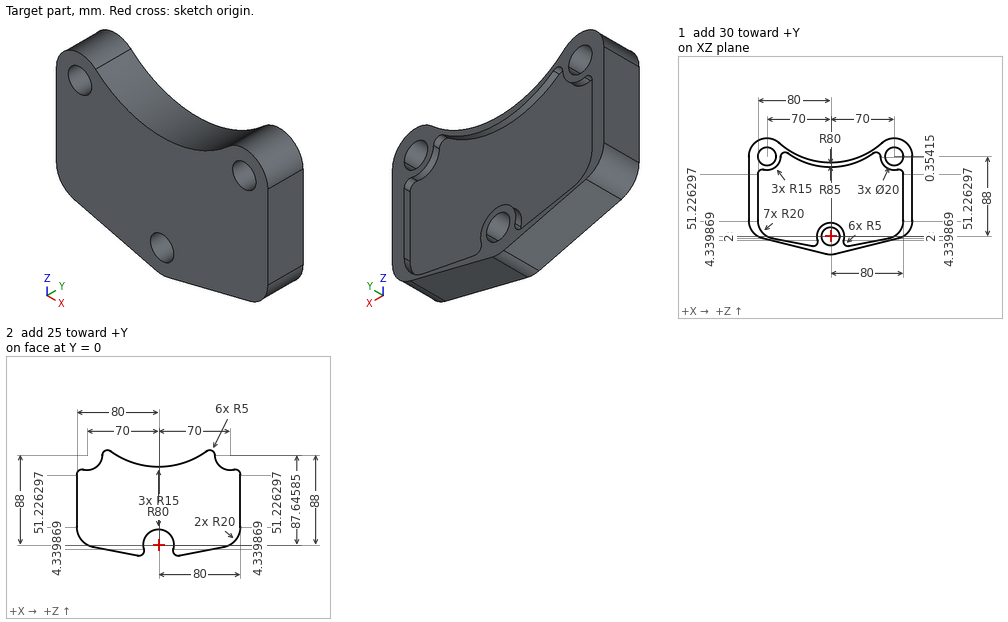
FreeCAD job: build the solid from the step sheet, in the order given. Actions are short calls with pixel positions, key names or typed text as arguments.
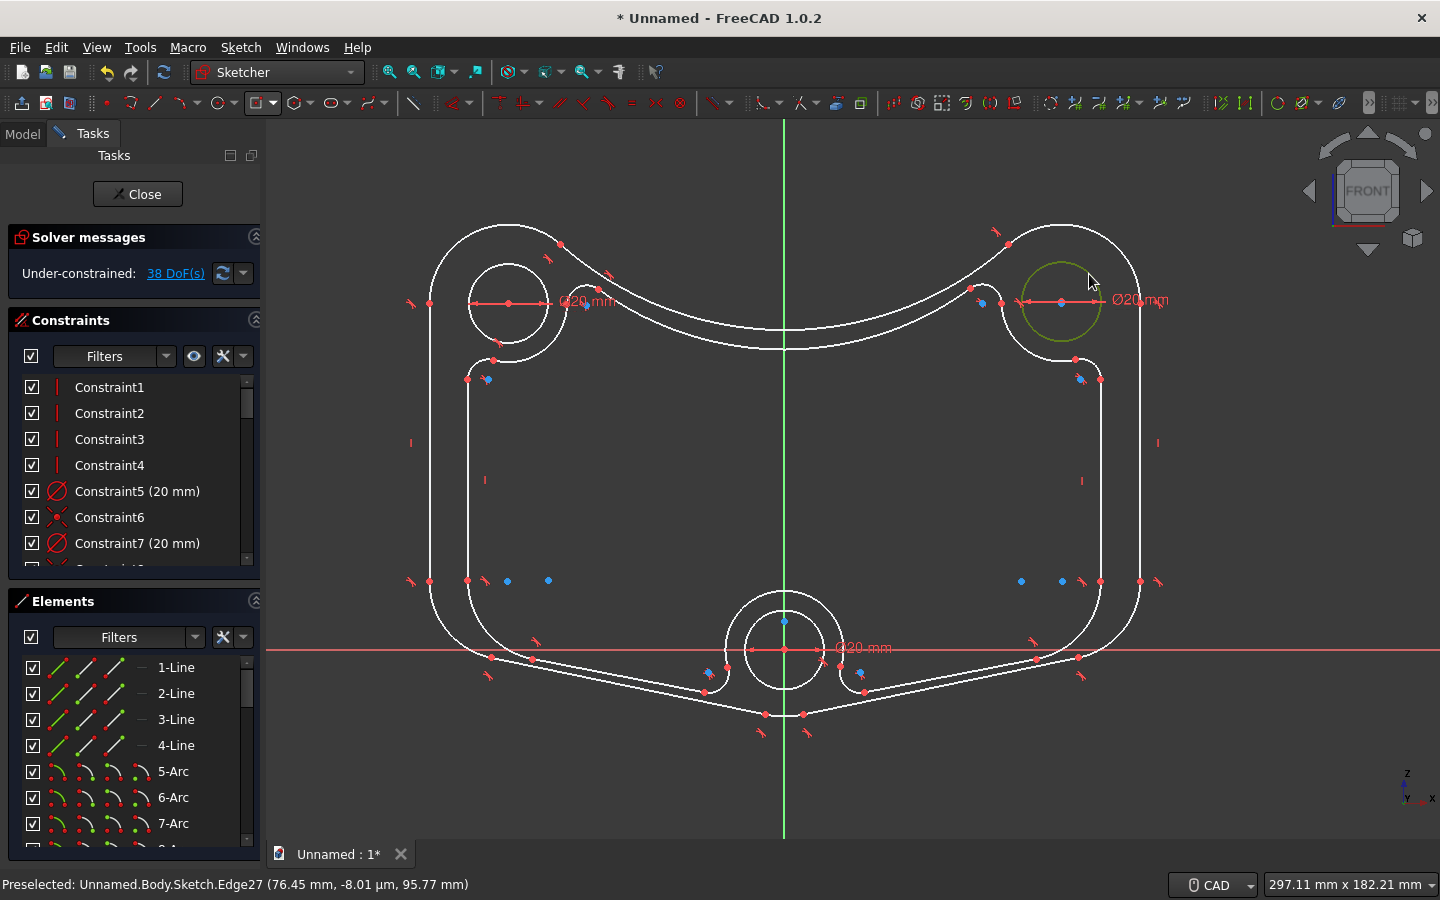
click(1122, 253)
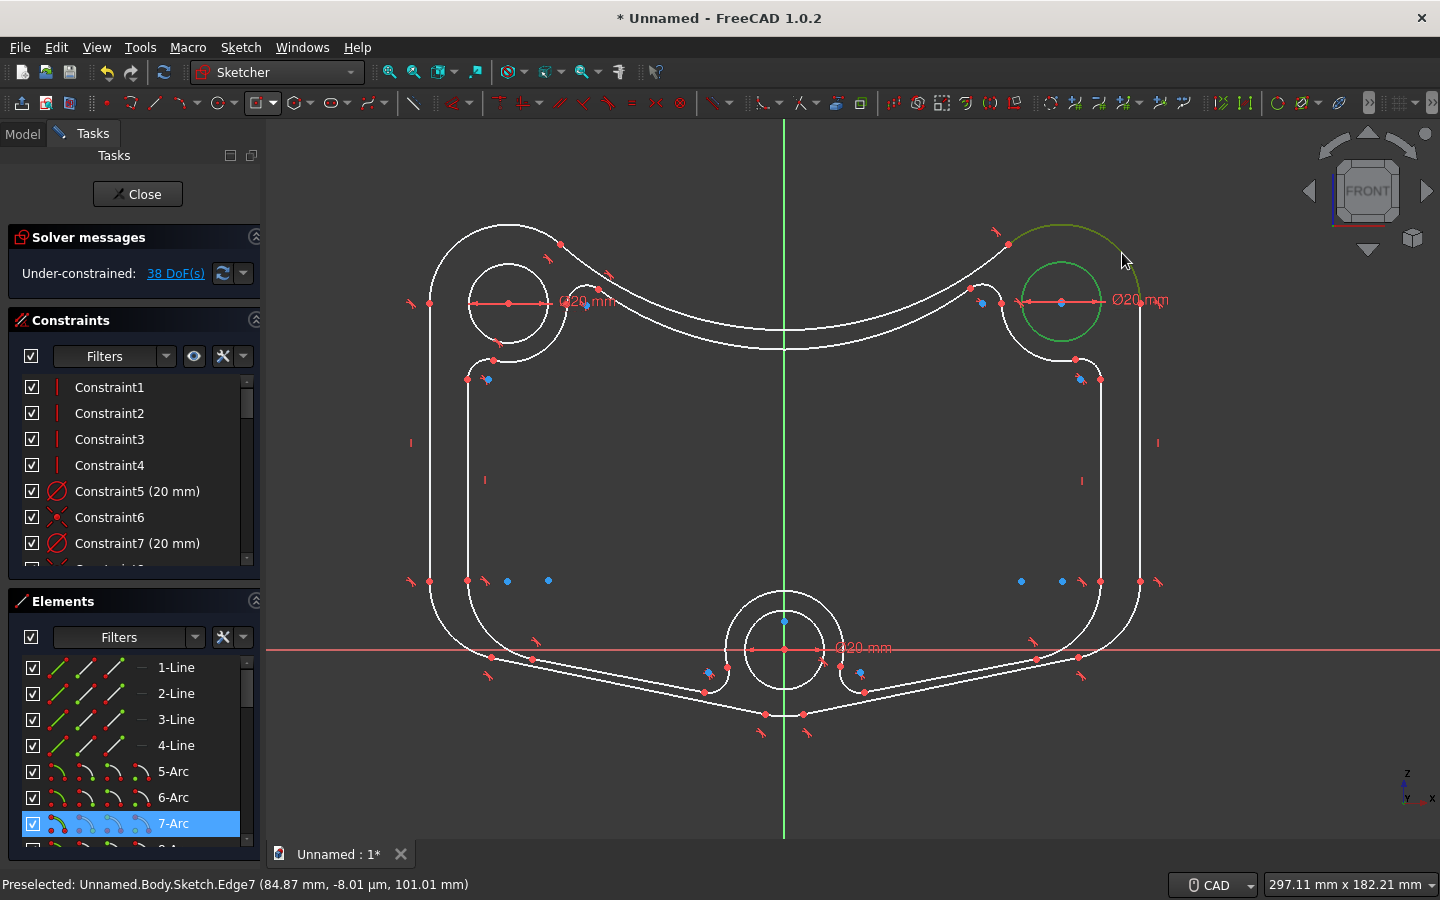
key(c)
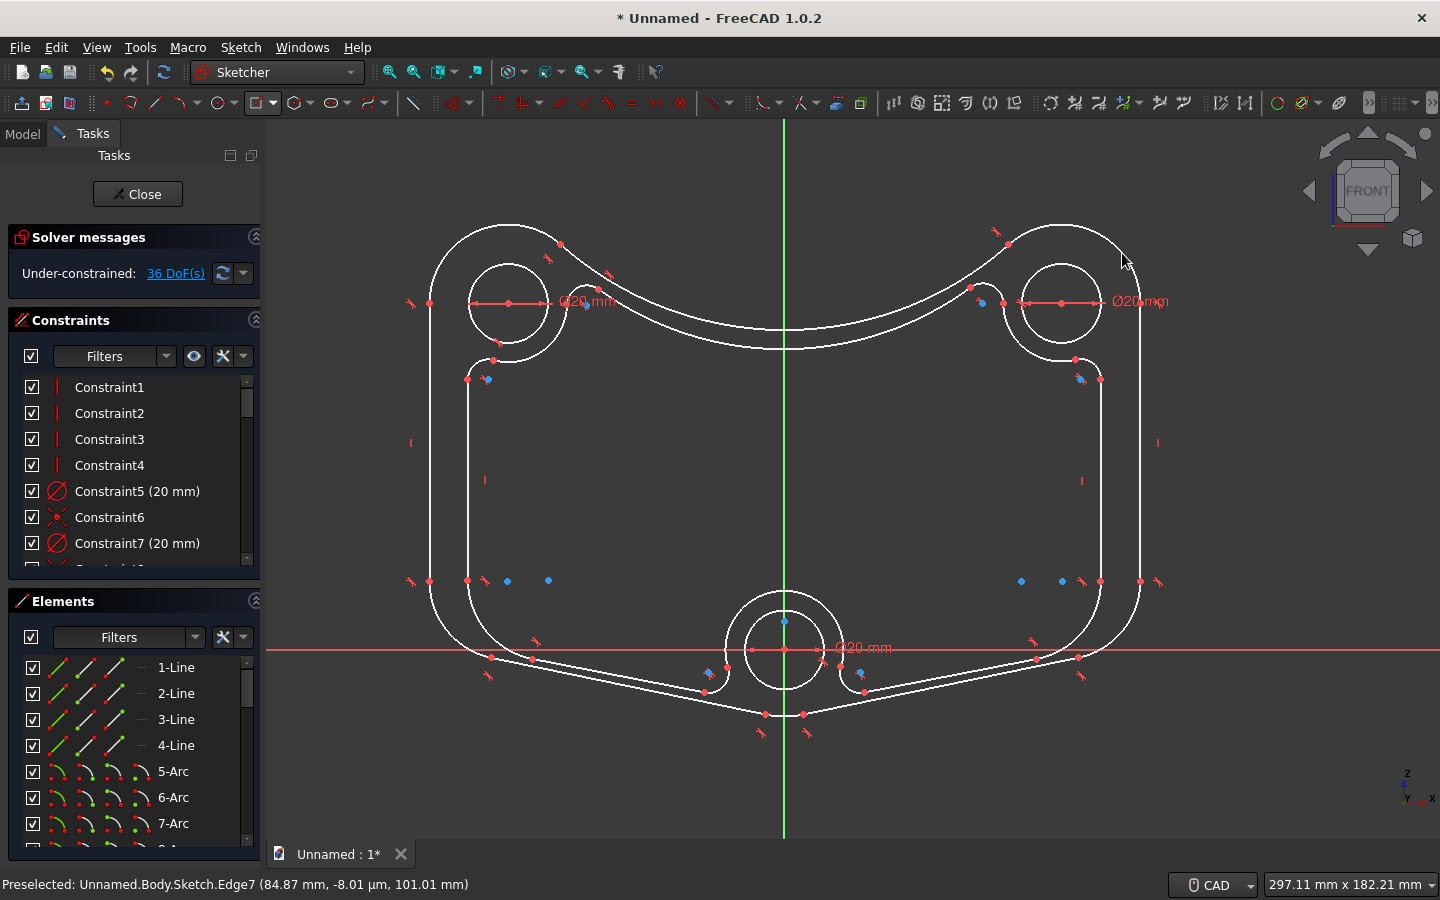
click(812, 622)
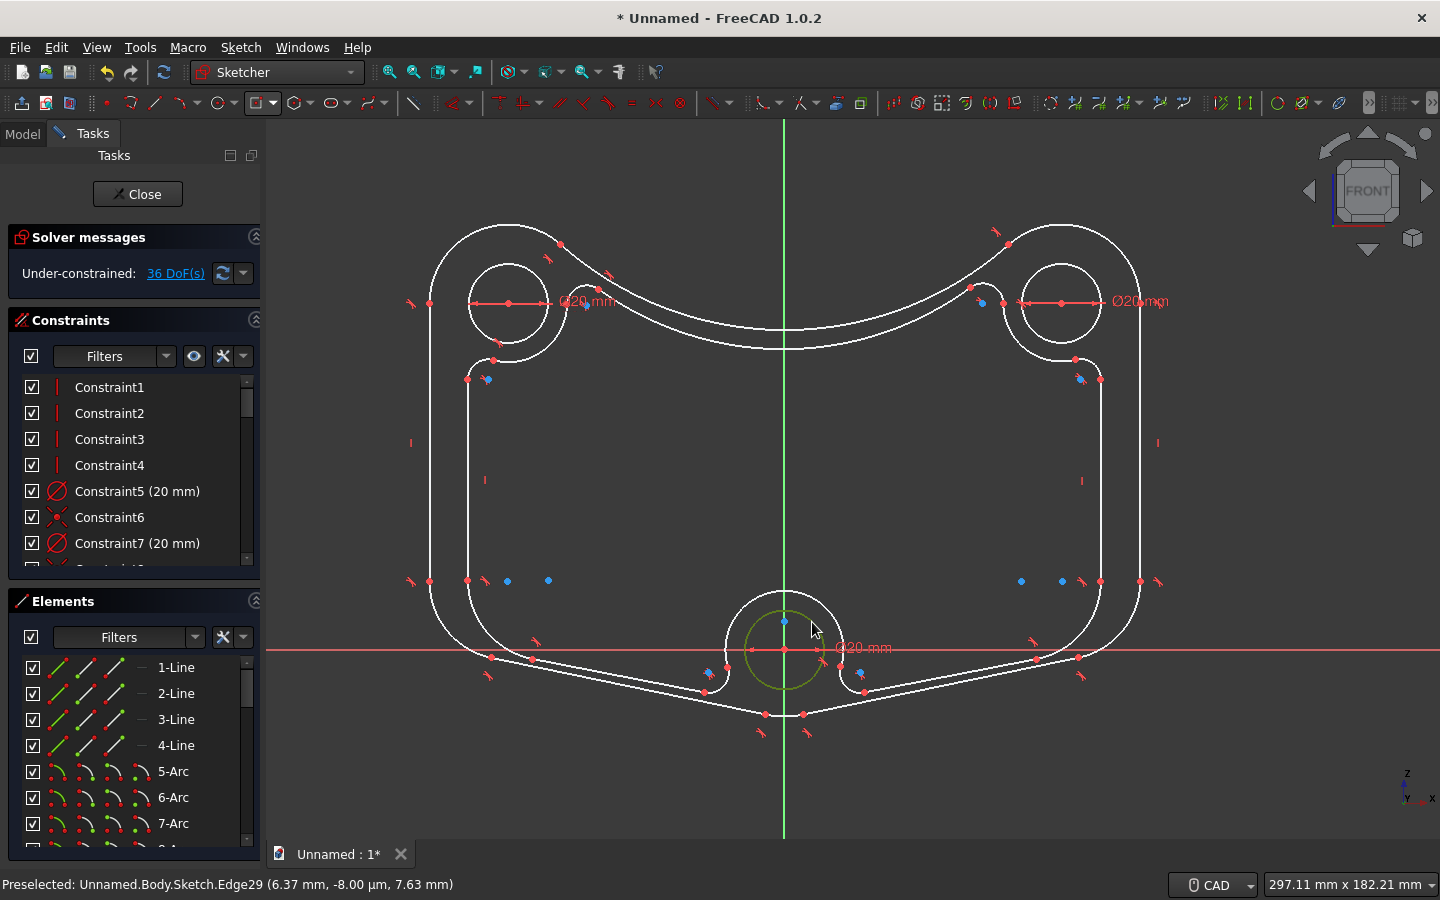
click(784, 716)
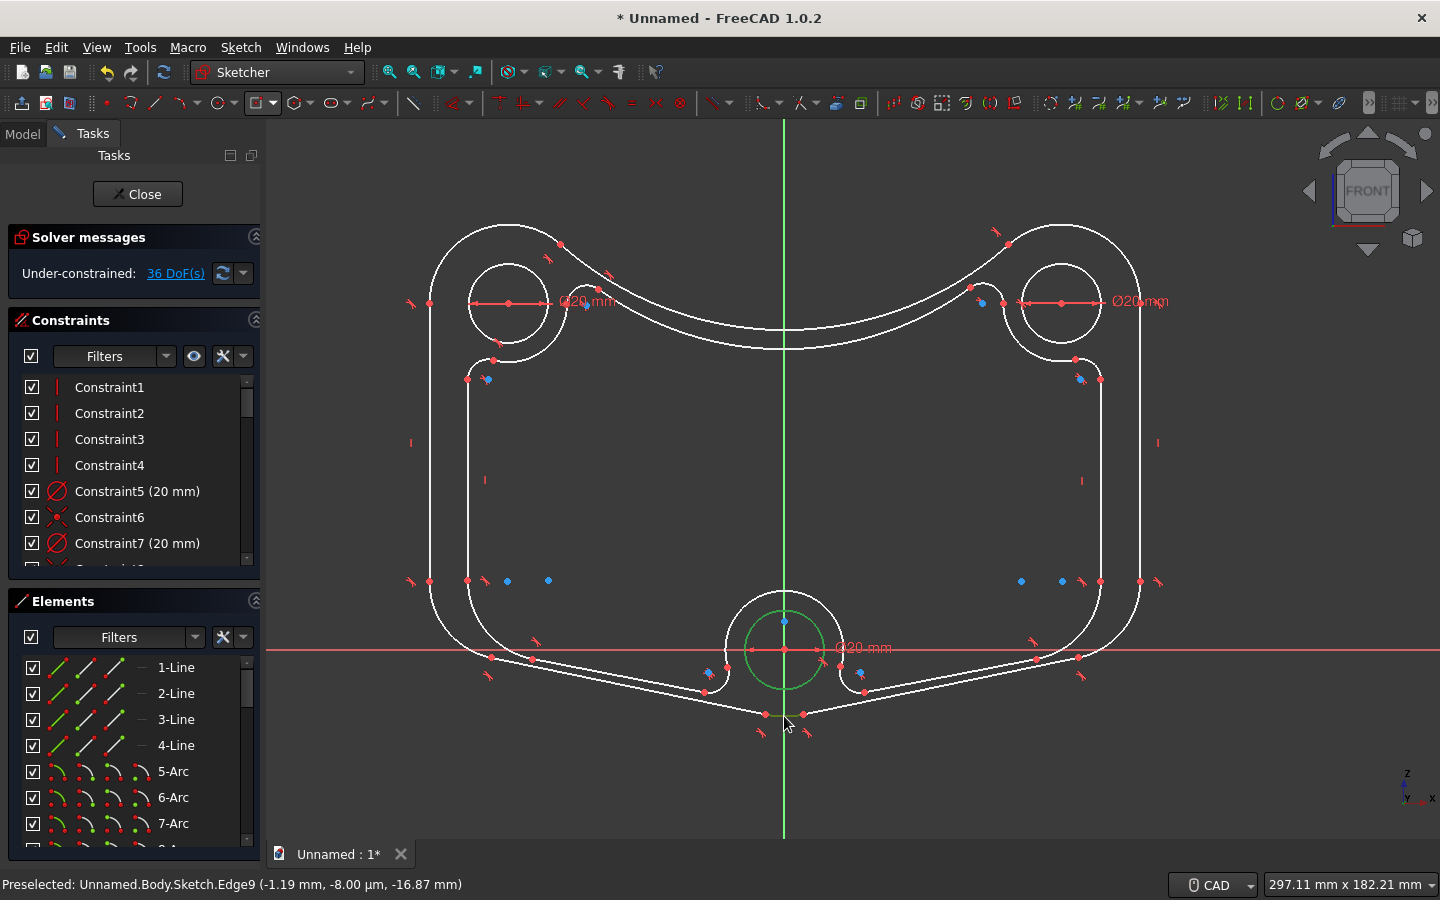
click(500, 104)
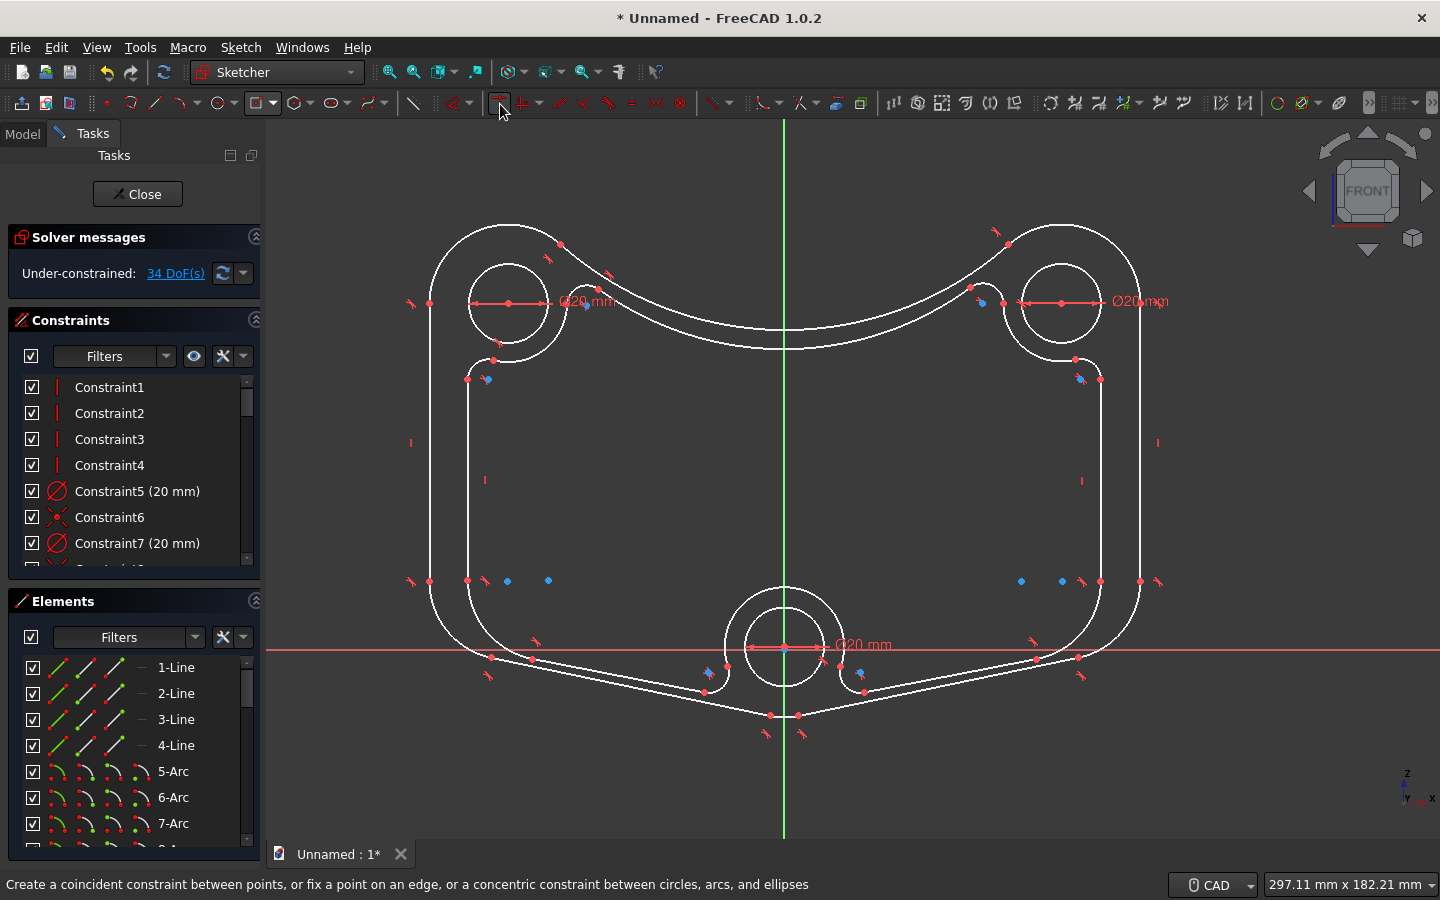
scroll(784, 648, up, 4)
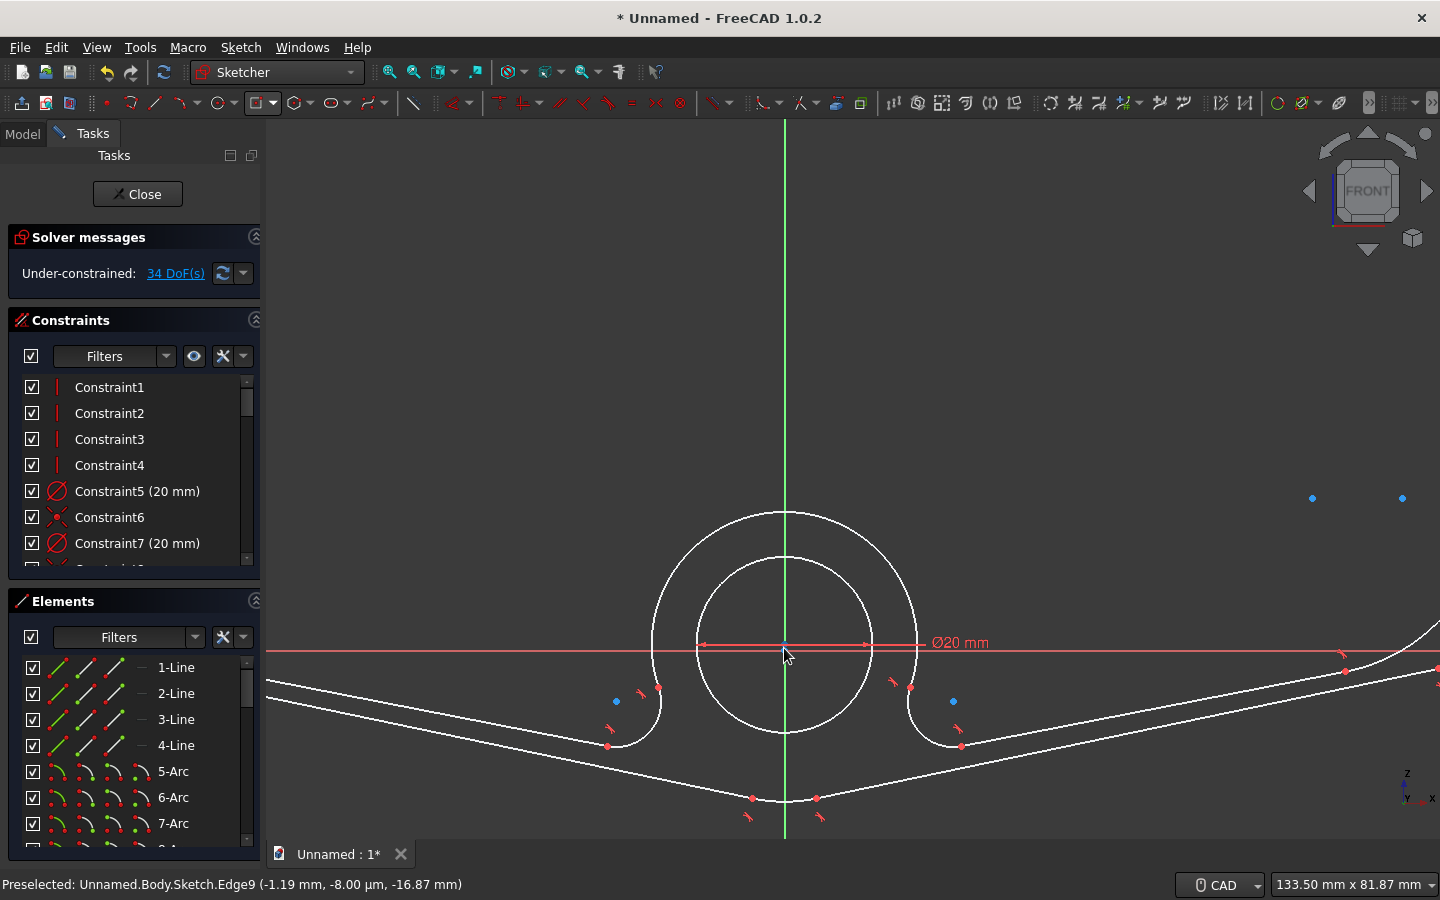
drag(774, 635, 795, 661)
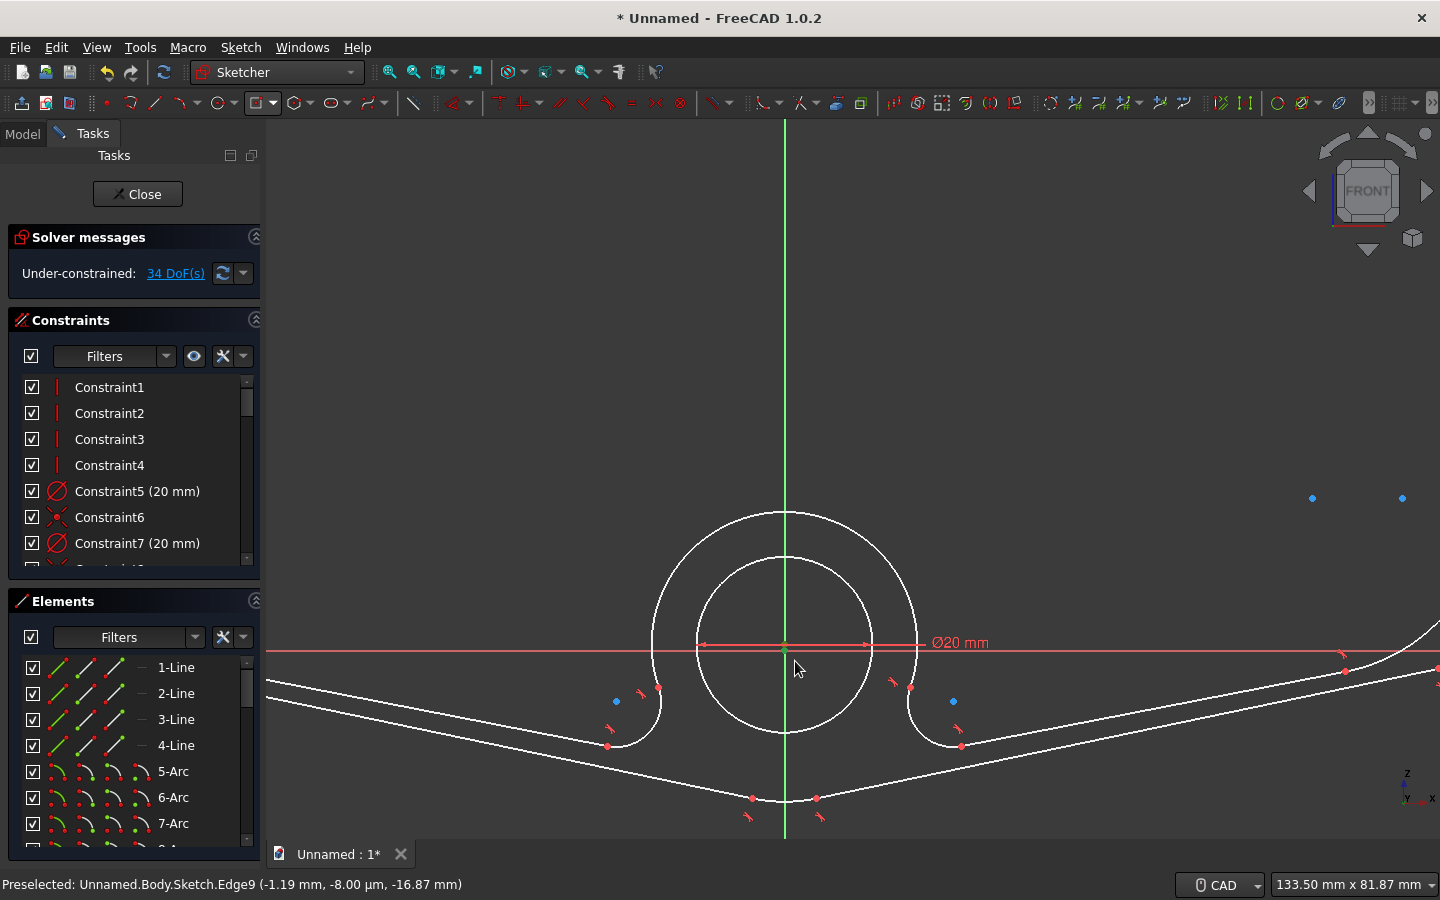
click(500, 104)